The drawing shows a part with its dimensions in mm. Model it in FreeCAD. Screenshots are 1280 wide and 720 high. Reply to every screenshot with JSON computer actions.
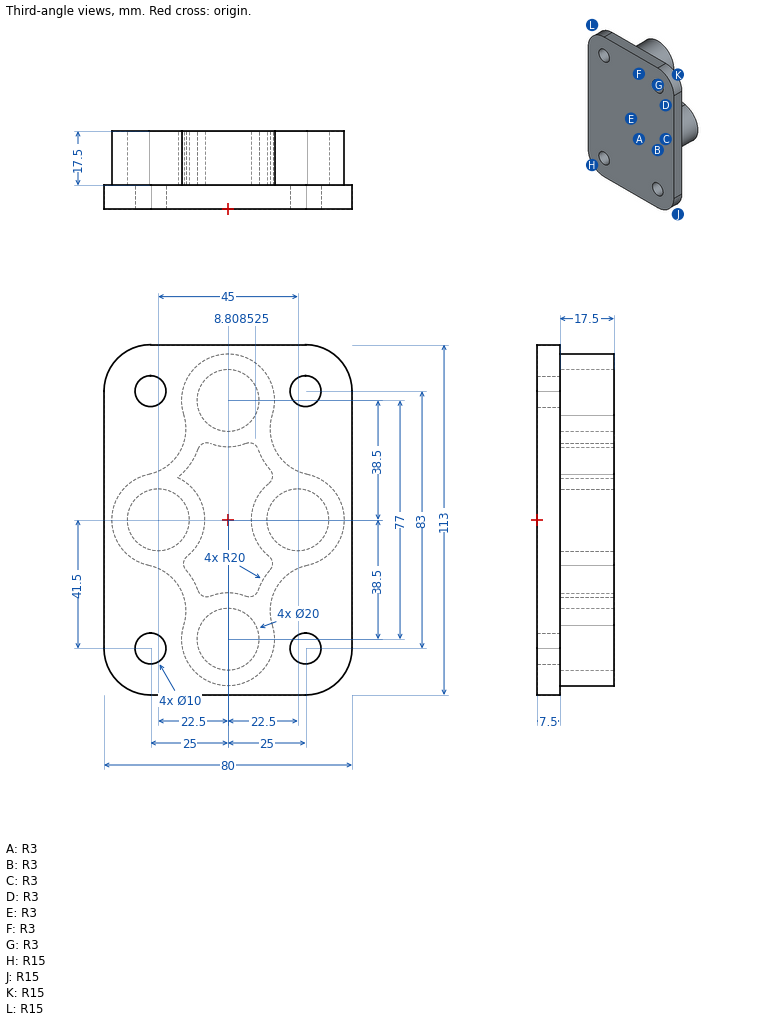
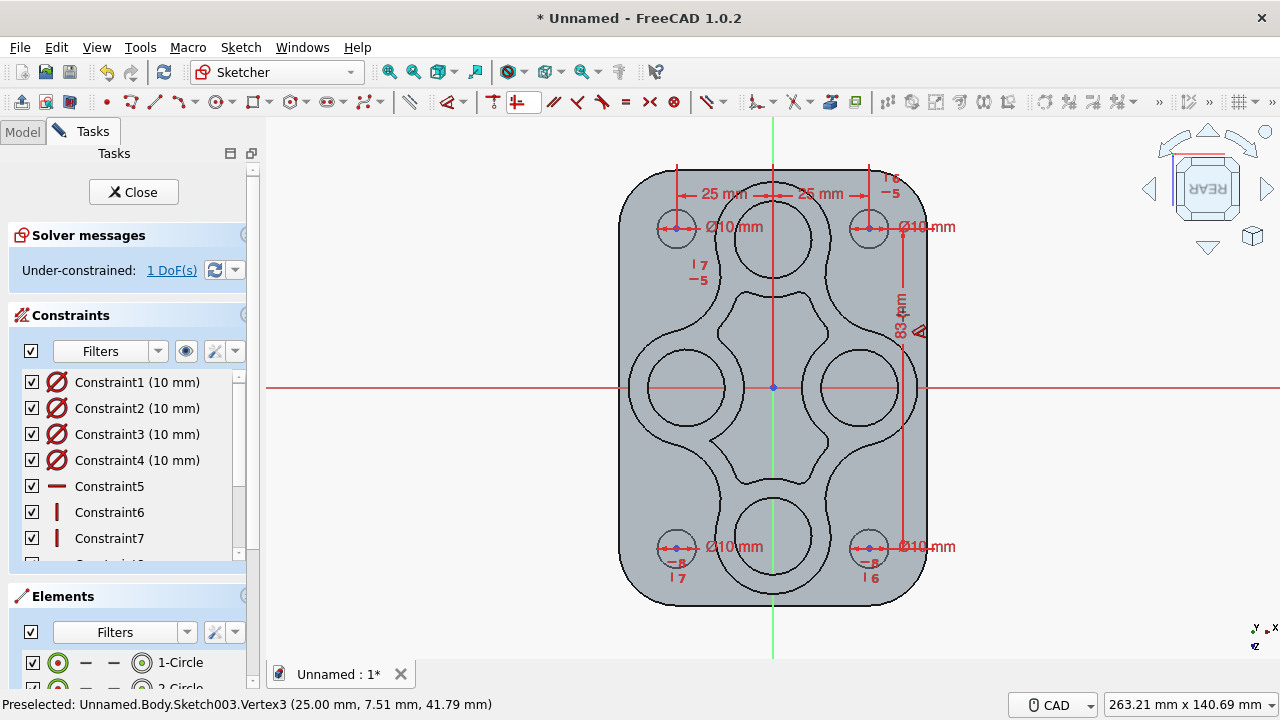
{"action": "left_click", "coordinate": [677, 229]}
{"action": "left_click", "coordinate": [643, 309]}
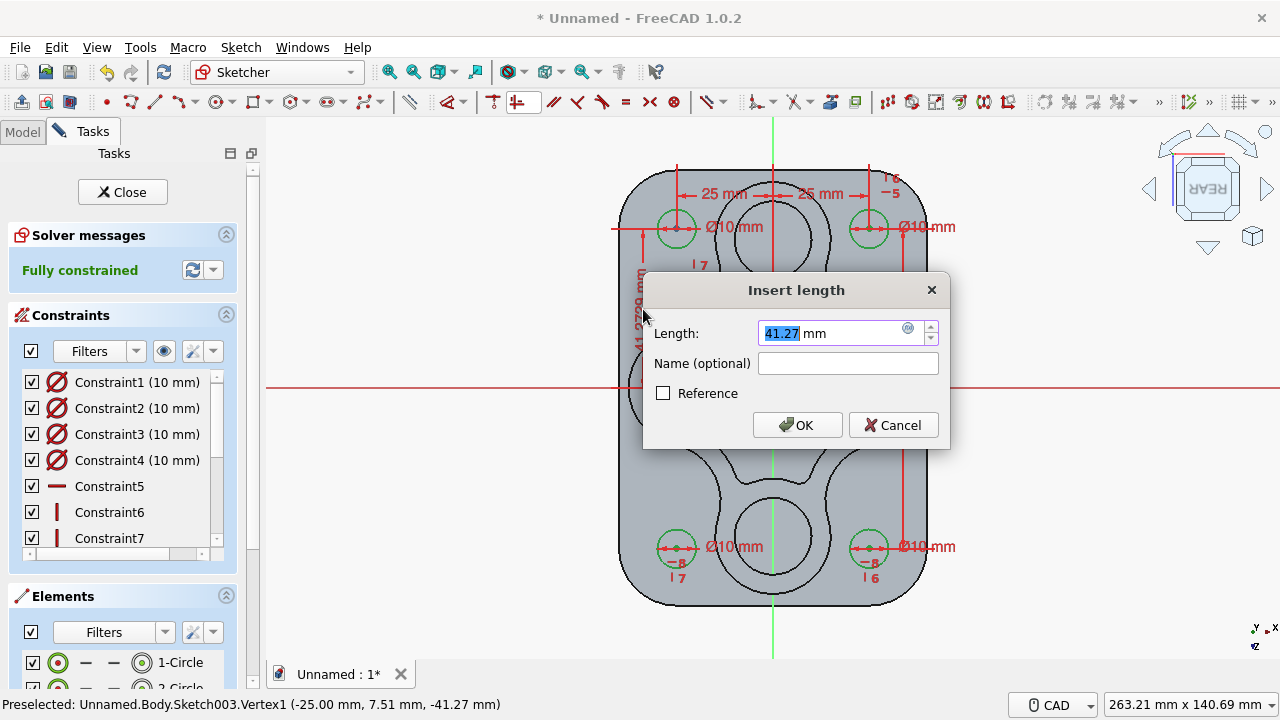
{"action": "type", "text": "41.5"}
{"action": "key", "text": "Return"}
{"action": "key", "text": "Escape"}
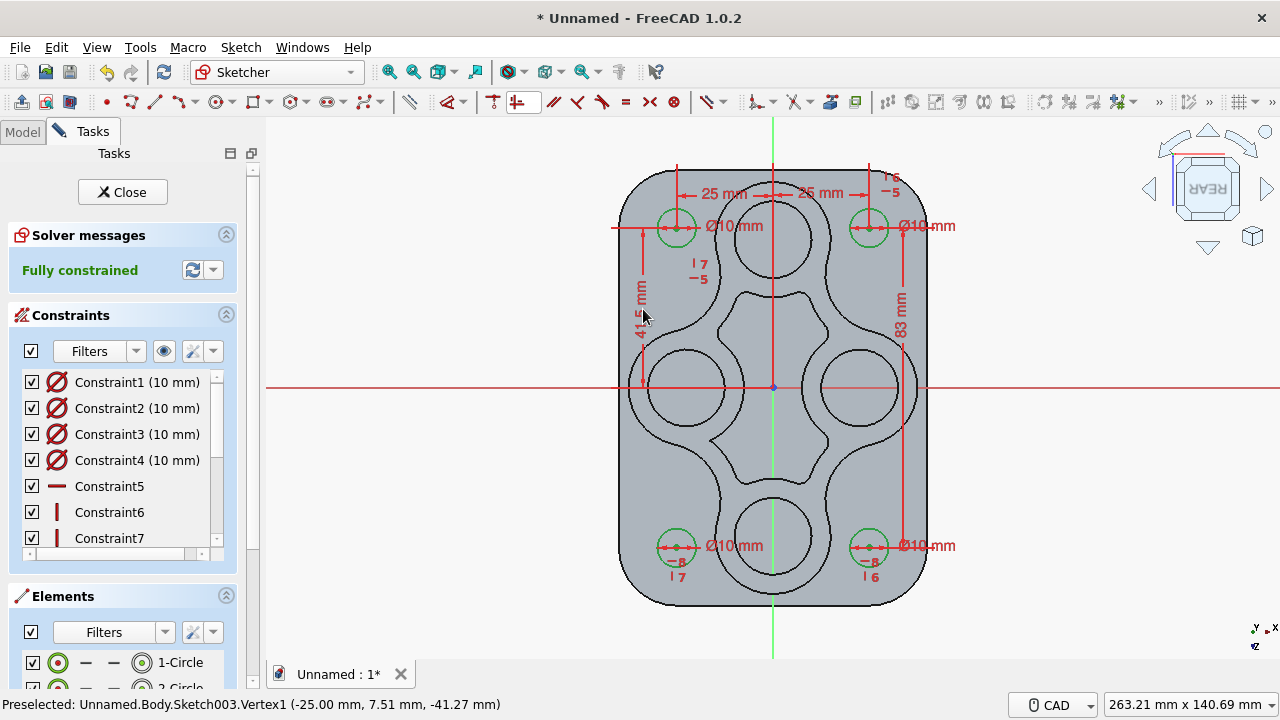
{"action": "left_click", "coordinate": [123, 192]}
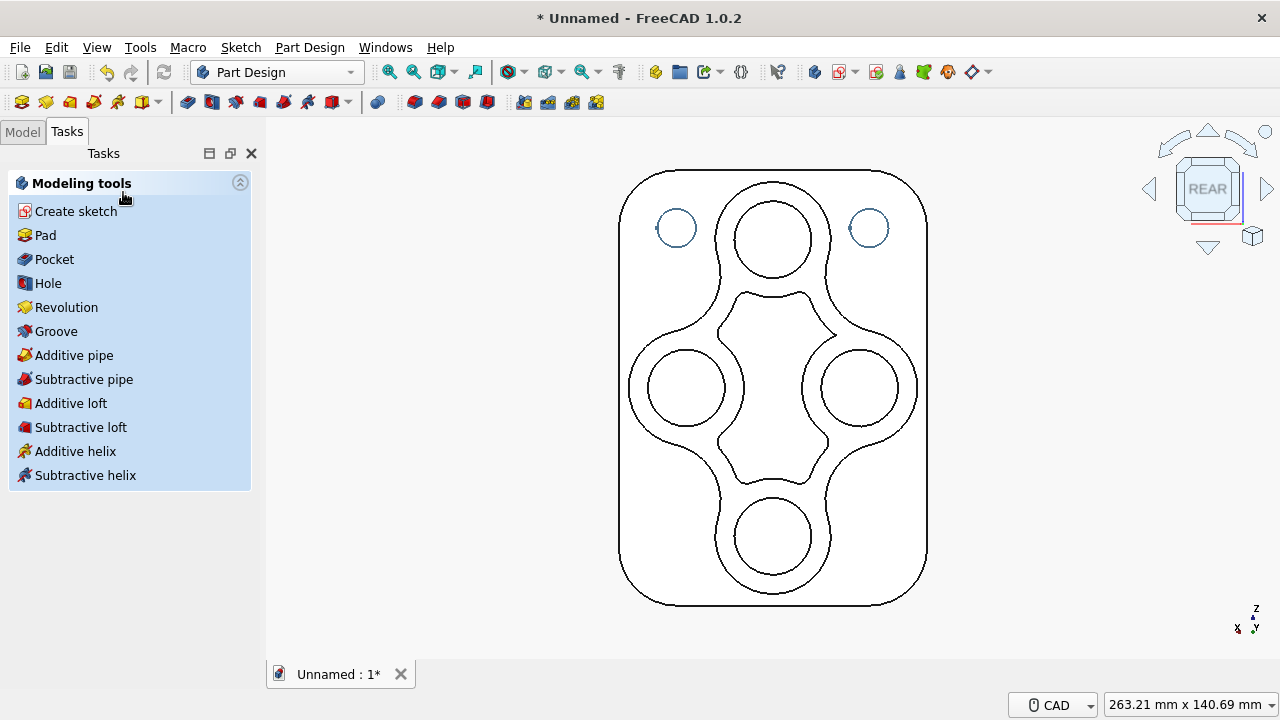
{"action": "left_click", "coordinate": [188, 102]}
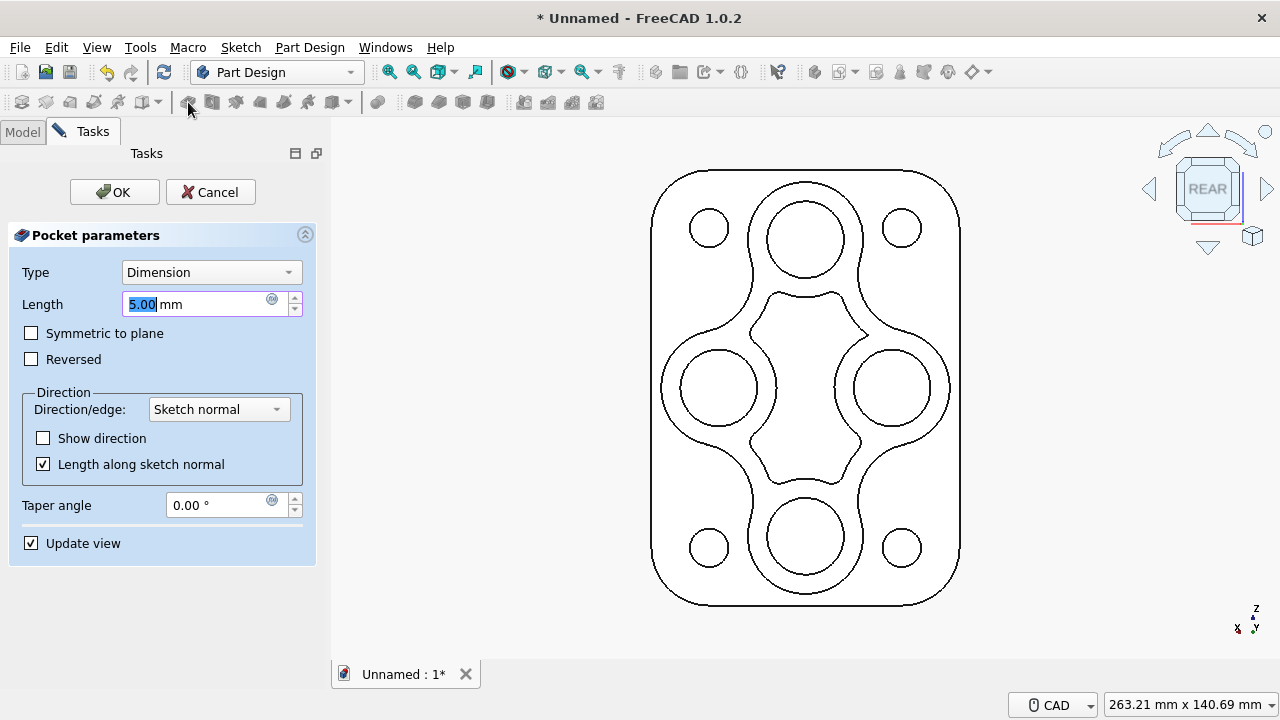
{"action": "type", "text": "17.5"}
{"action": "key", "text": "Tab"}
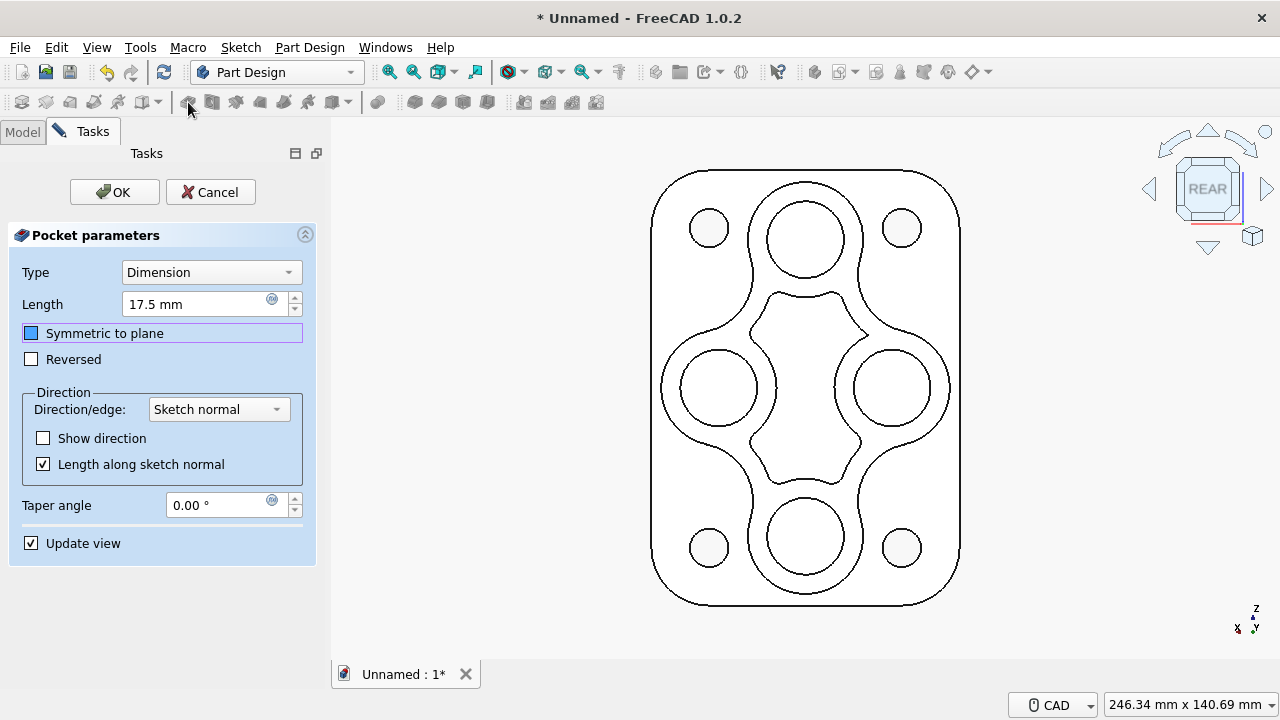
{"action": "left_click", "coordinate": [115, 192]}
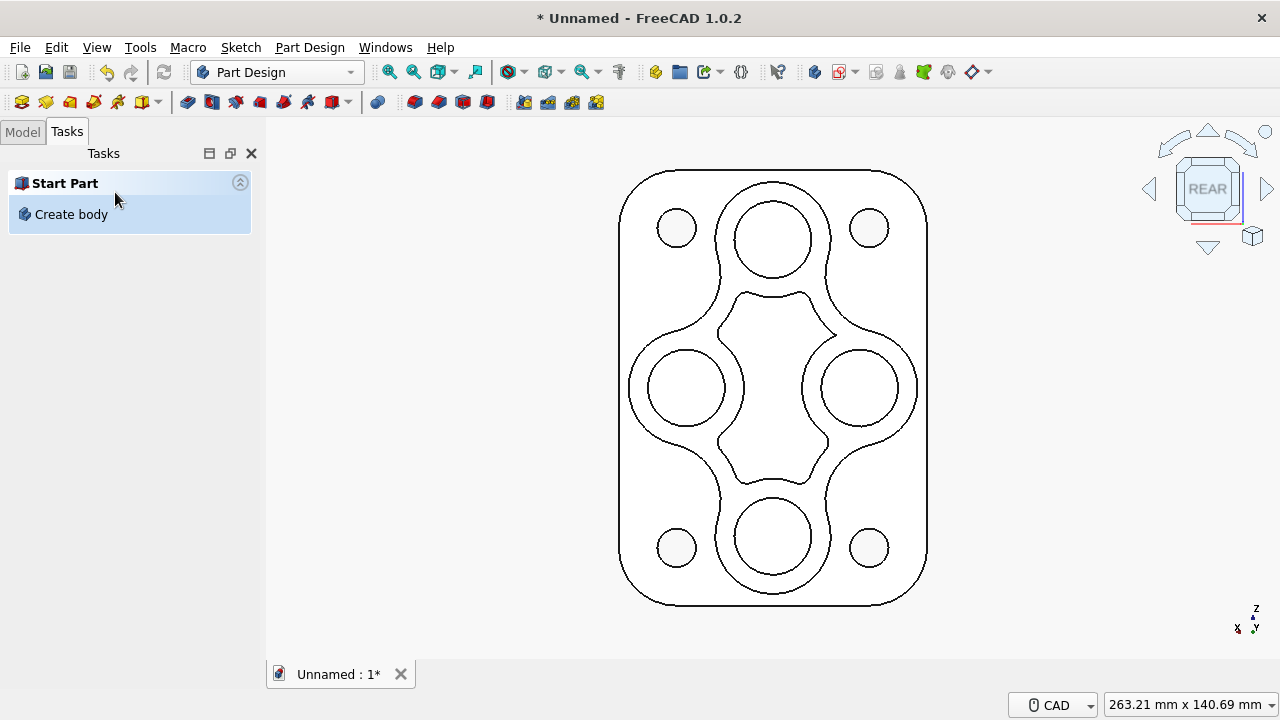
{"action": "key", "text": "0"}